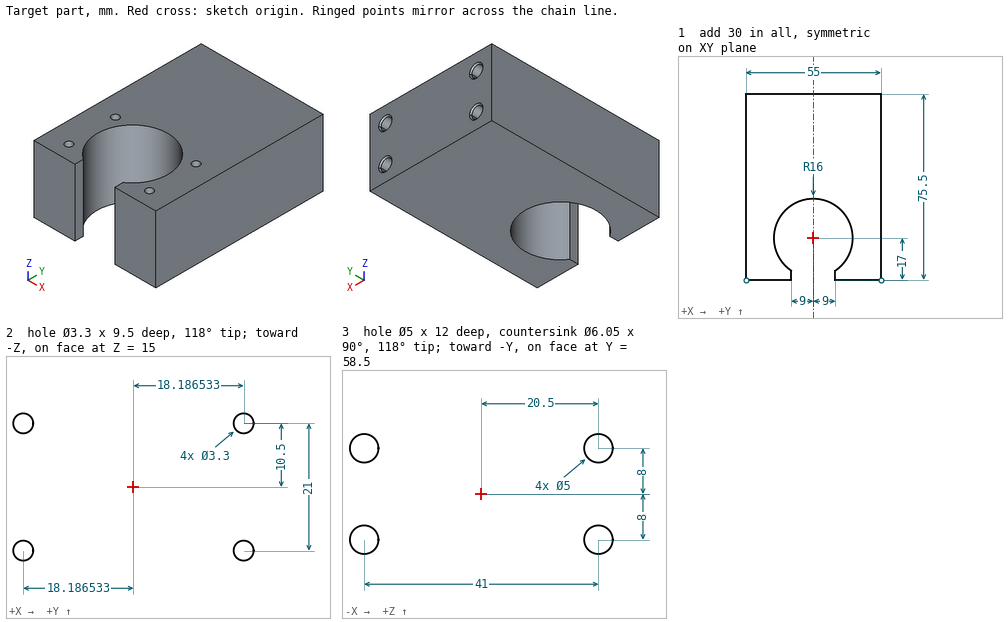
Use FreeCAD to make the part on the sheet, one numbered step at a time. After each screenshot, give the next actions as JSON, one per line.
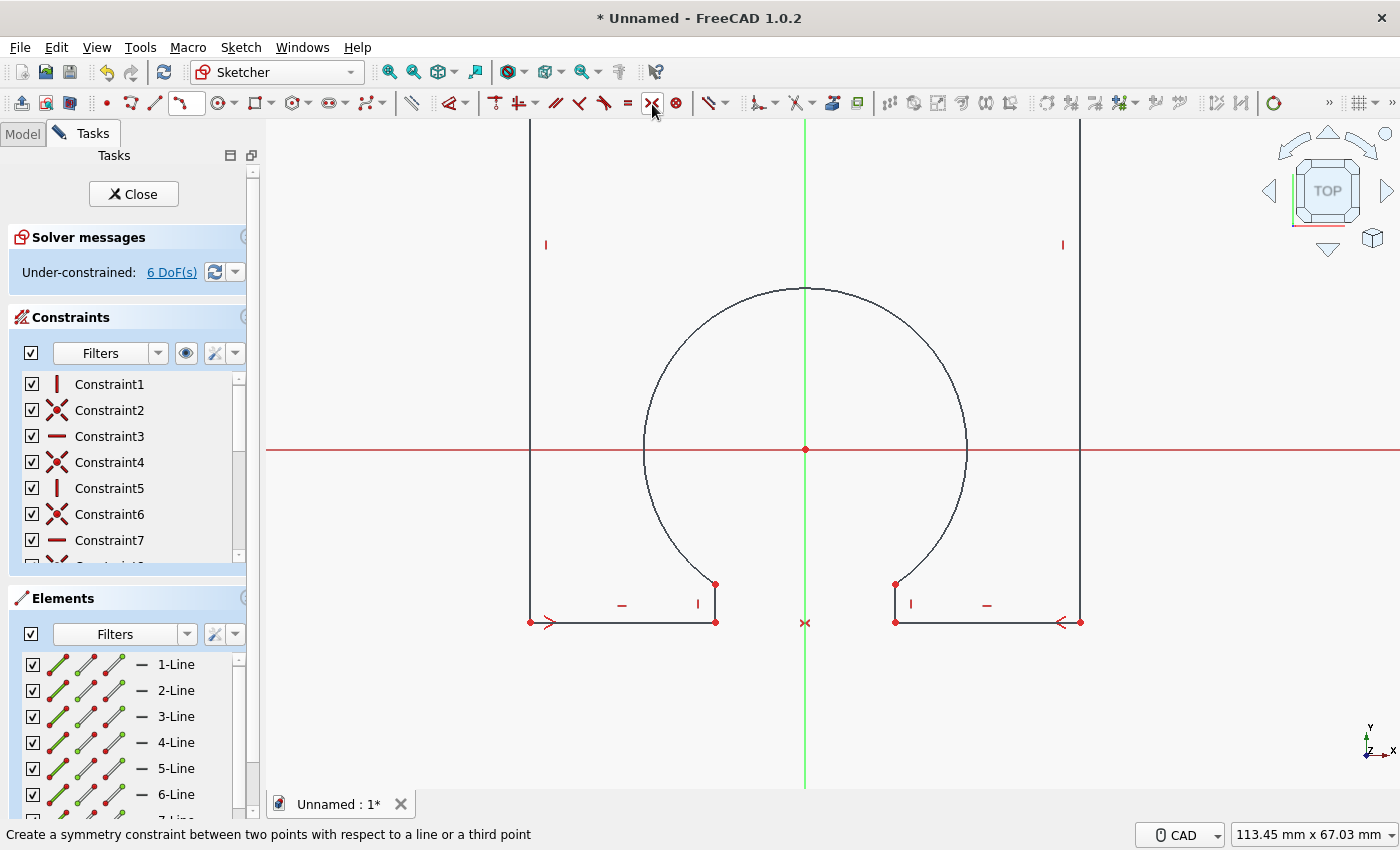
{"action": "left_click", "coordinate": [450, 104]}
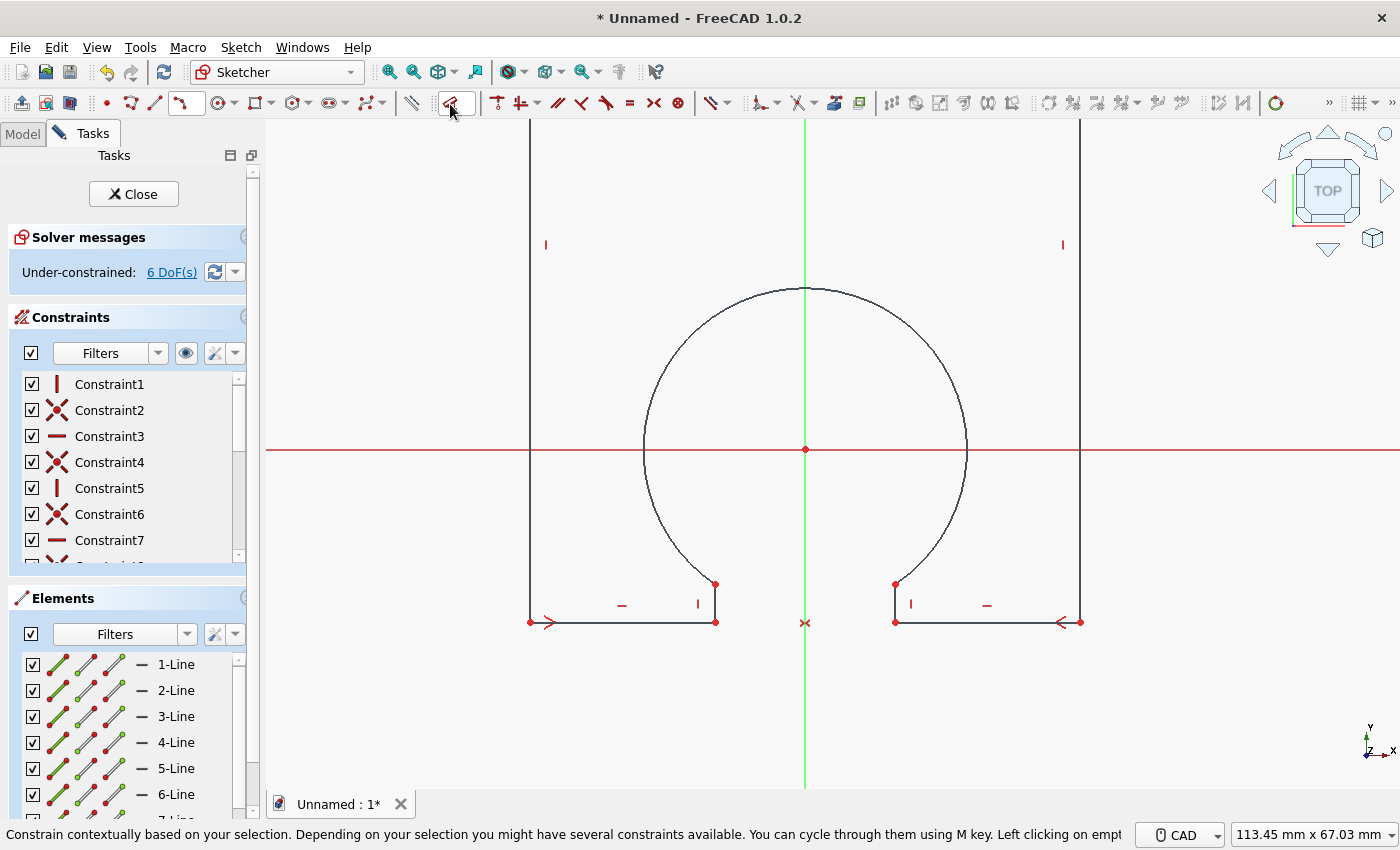
{"action": "left_click", "coordinate": [943, 365]}
{"action": "left_click", "coordinate": [970, 348]}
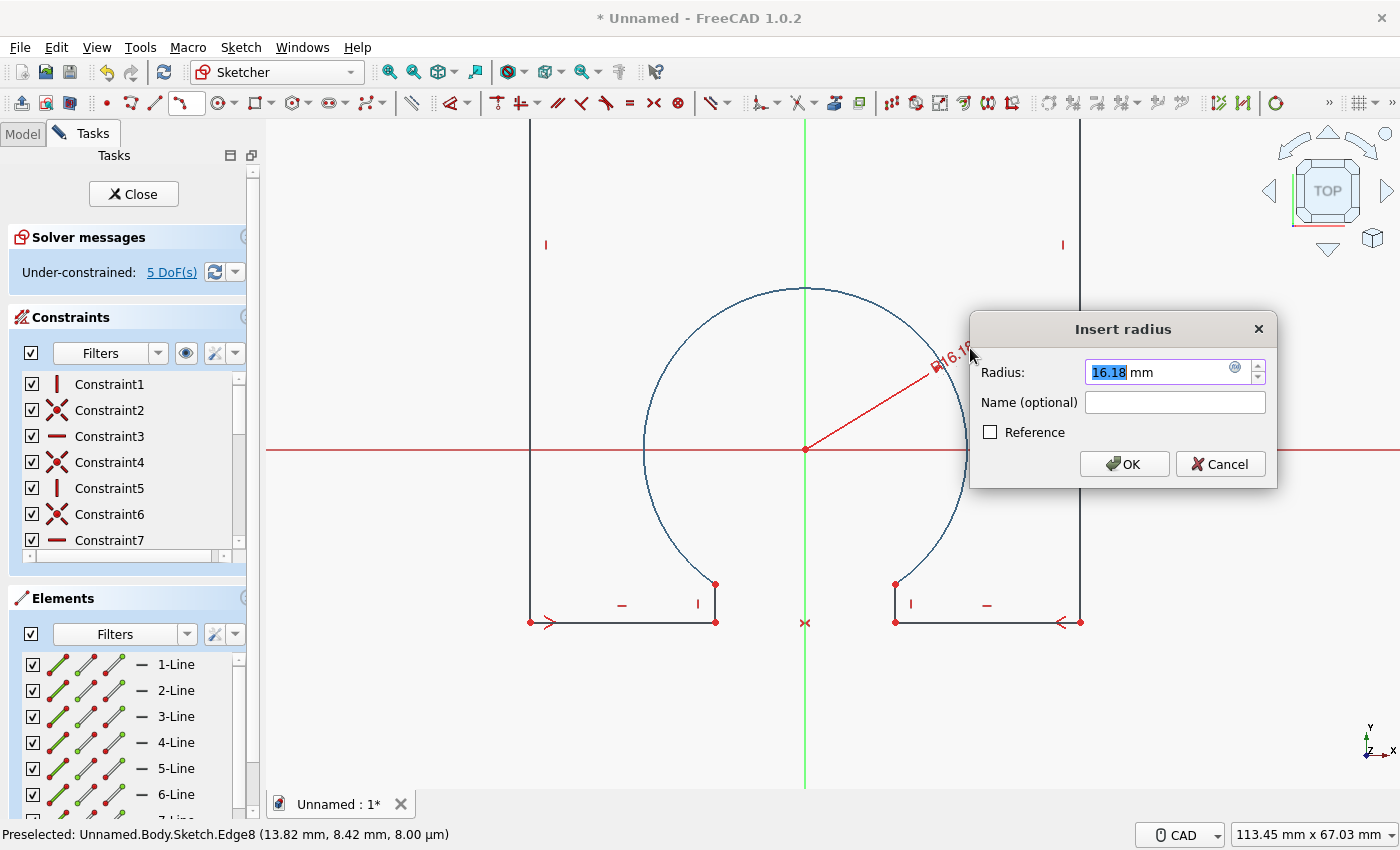
{"action": "type", "text": "16"}
{"action": "key", "text": "Return"}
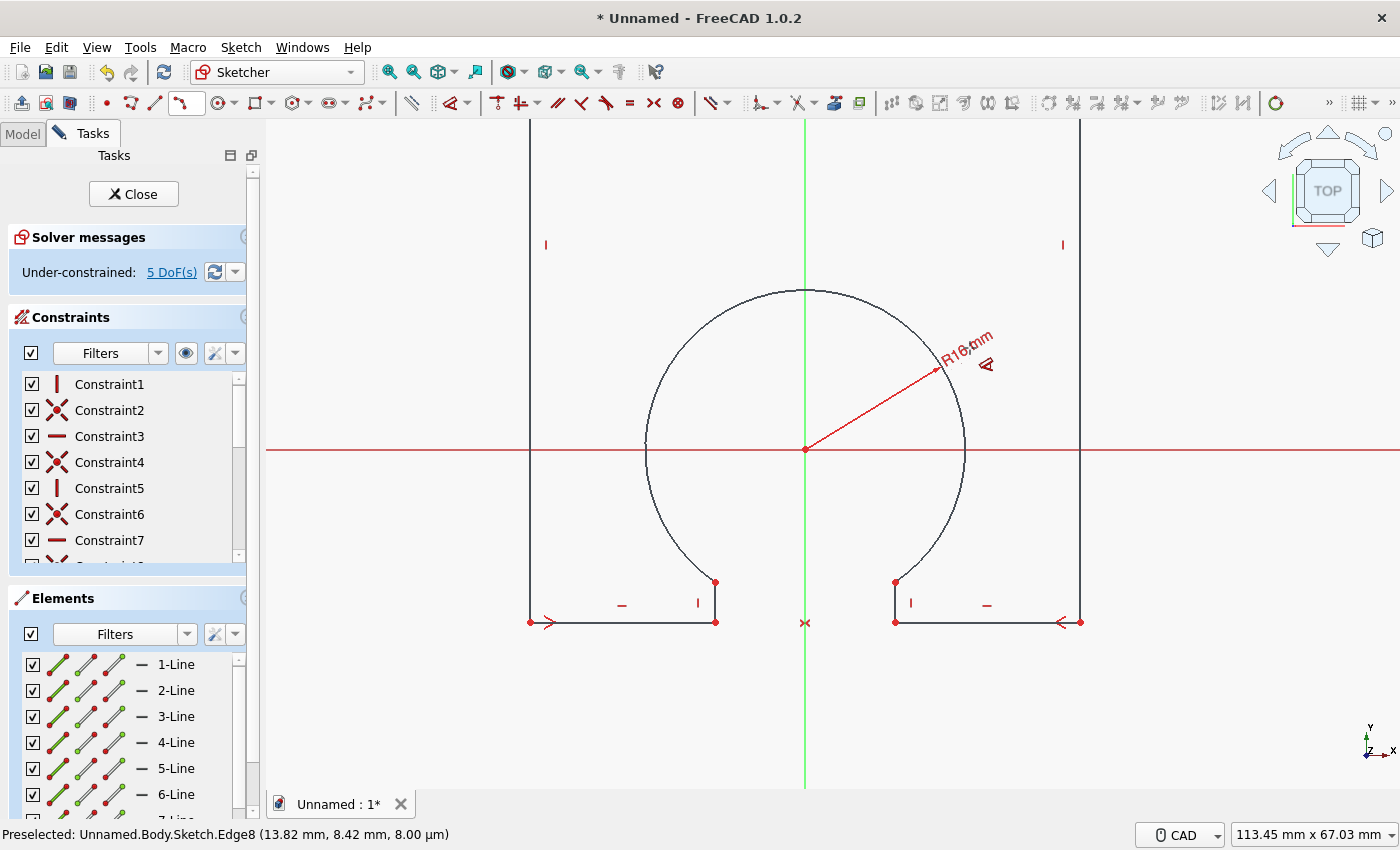
{"action": "scroll", "coordinate": [715, 711], "scroll_direction": "down", "scroll_amount": 3}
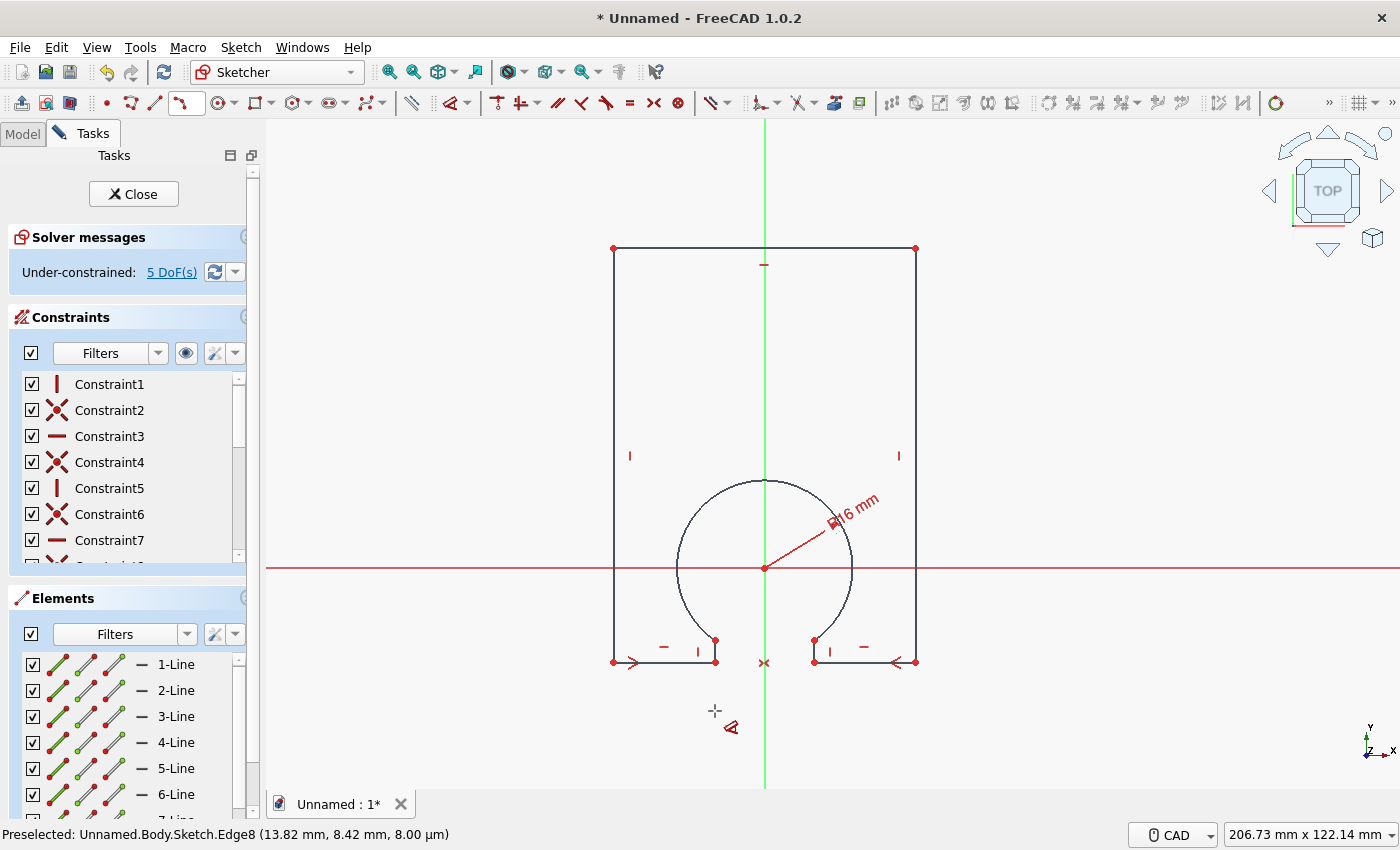
{"action": "left_click", "coordinate": [825, 248]}
{"action": "left_click", "coordinate": [695, 214]}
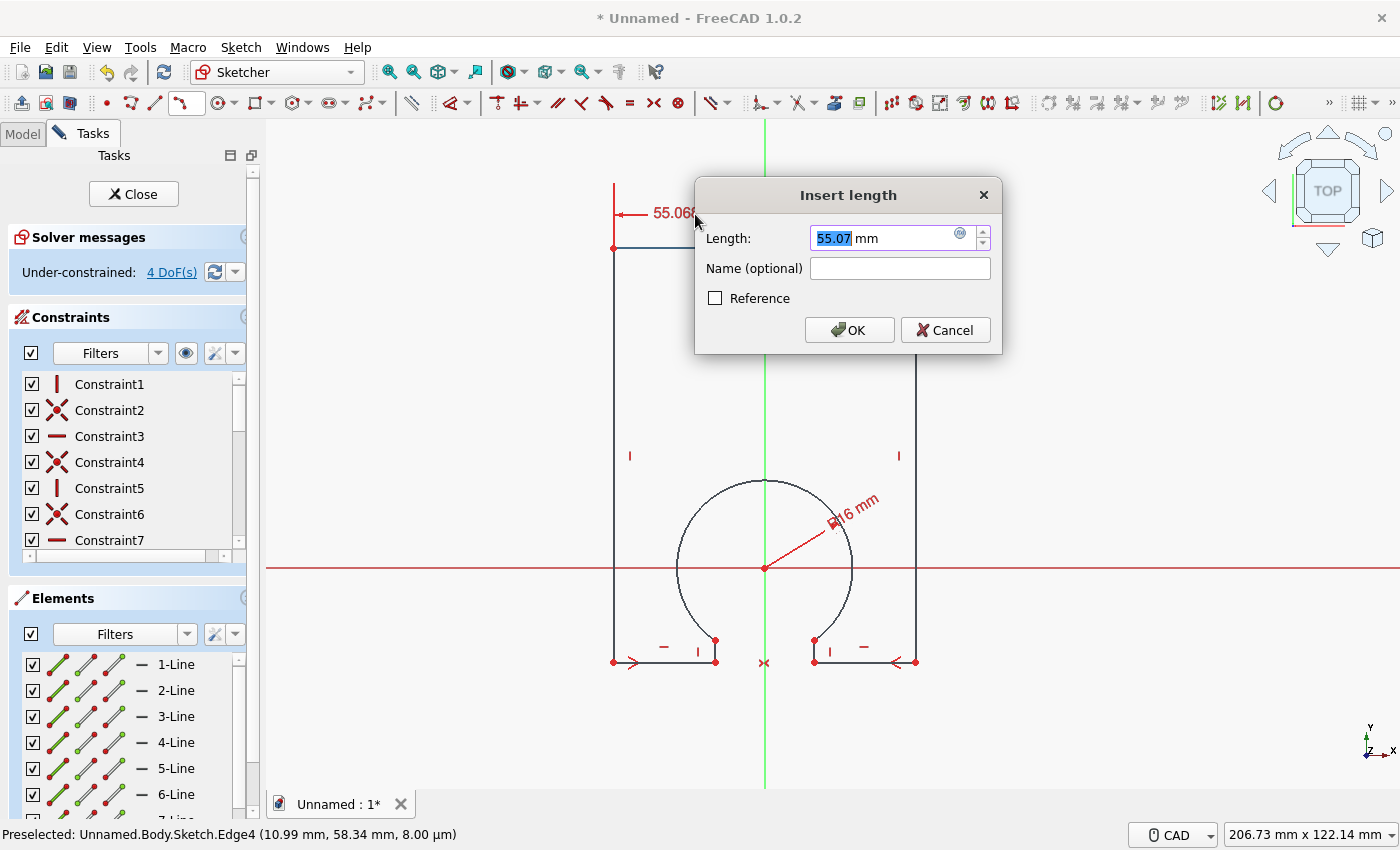
{"action": "type", "text": "55"}
{"action": "key", "text": "Return"}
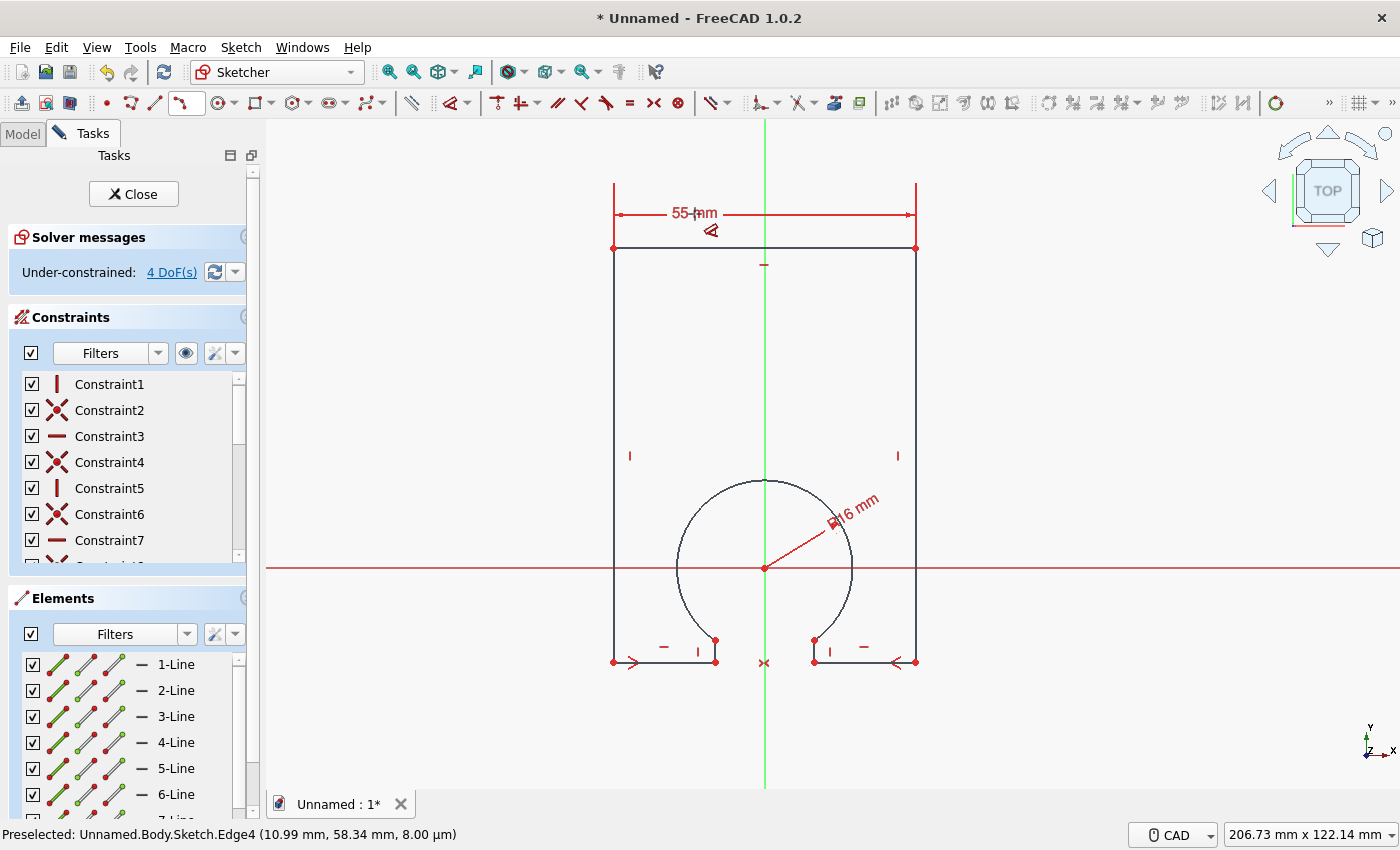
{"action": "left_click", "coordinate": [814, 641]}
{"action": "left_click", "coordinate": [789, 675]}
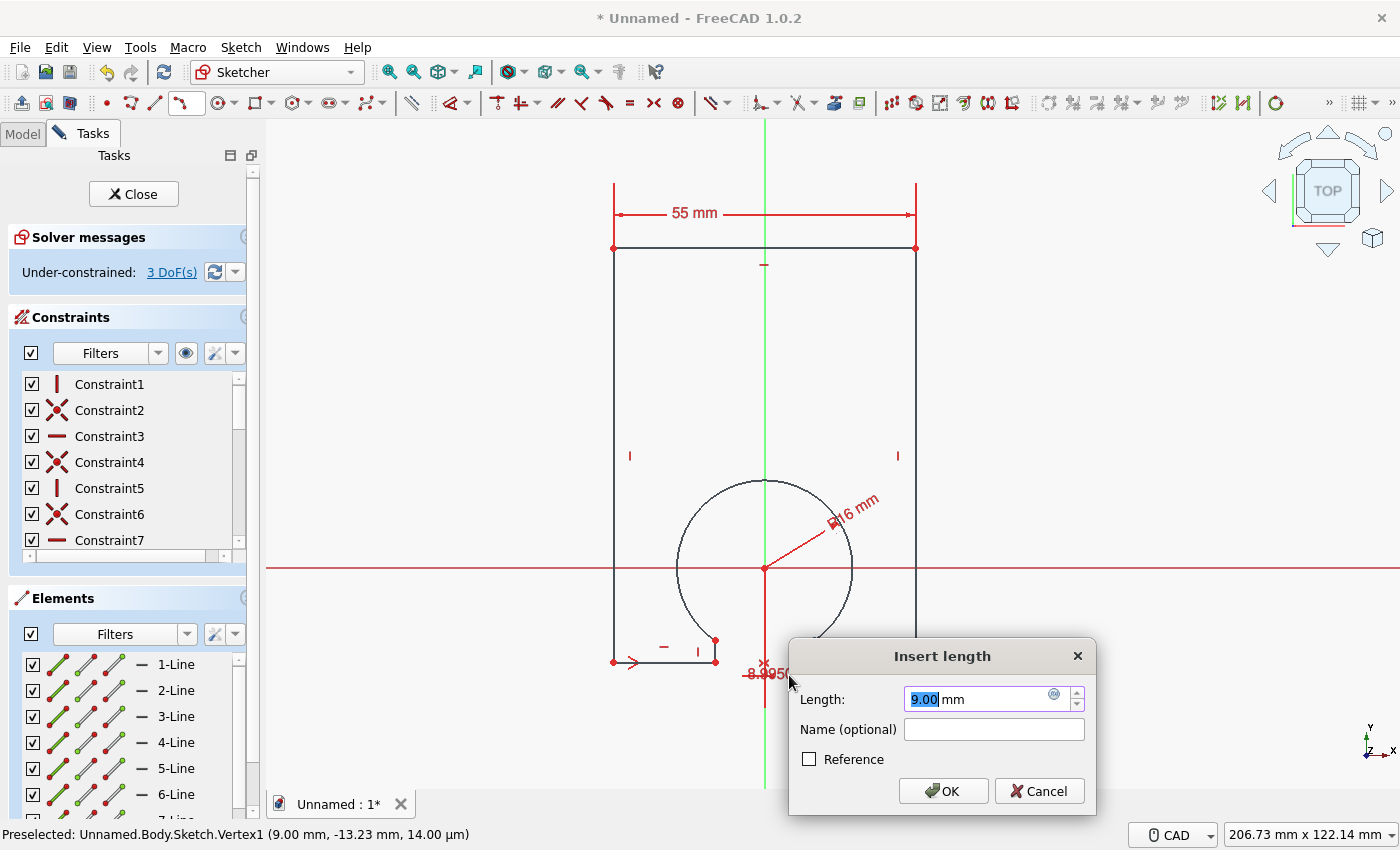
{"action": "type", "text": "9"}
{"action": "key", "text": "Return"}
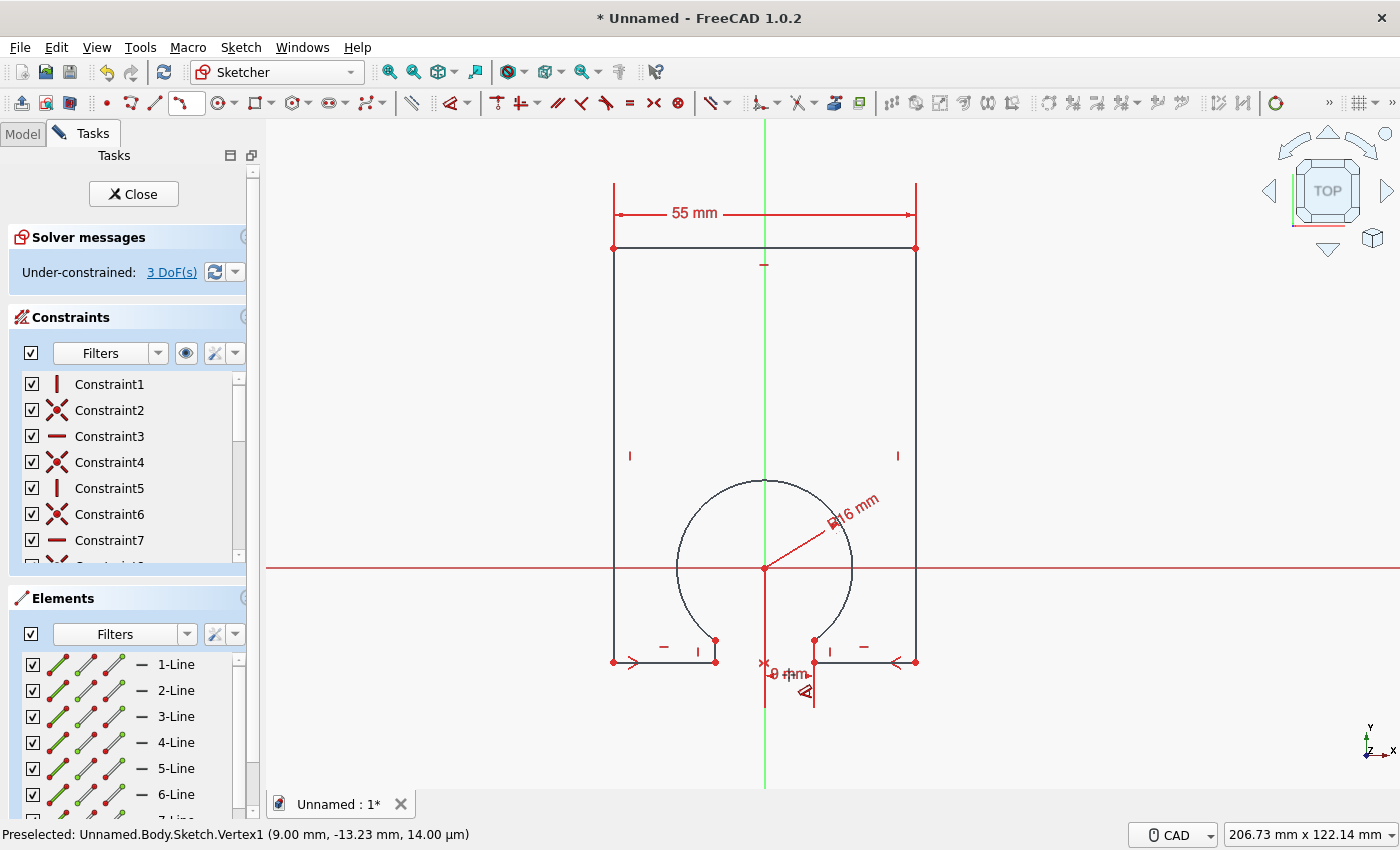
{"action": "left_click", "coordinate": [715, 663]}
{"action": "left_click", "coordinate": [740, 697]}